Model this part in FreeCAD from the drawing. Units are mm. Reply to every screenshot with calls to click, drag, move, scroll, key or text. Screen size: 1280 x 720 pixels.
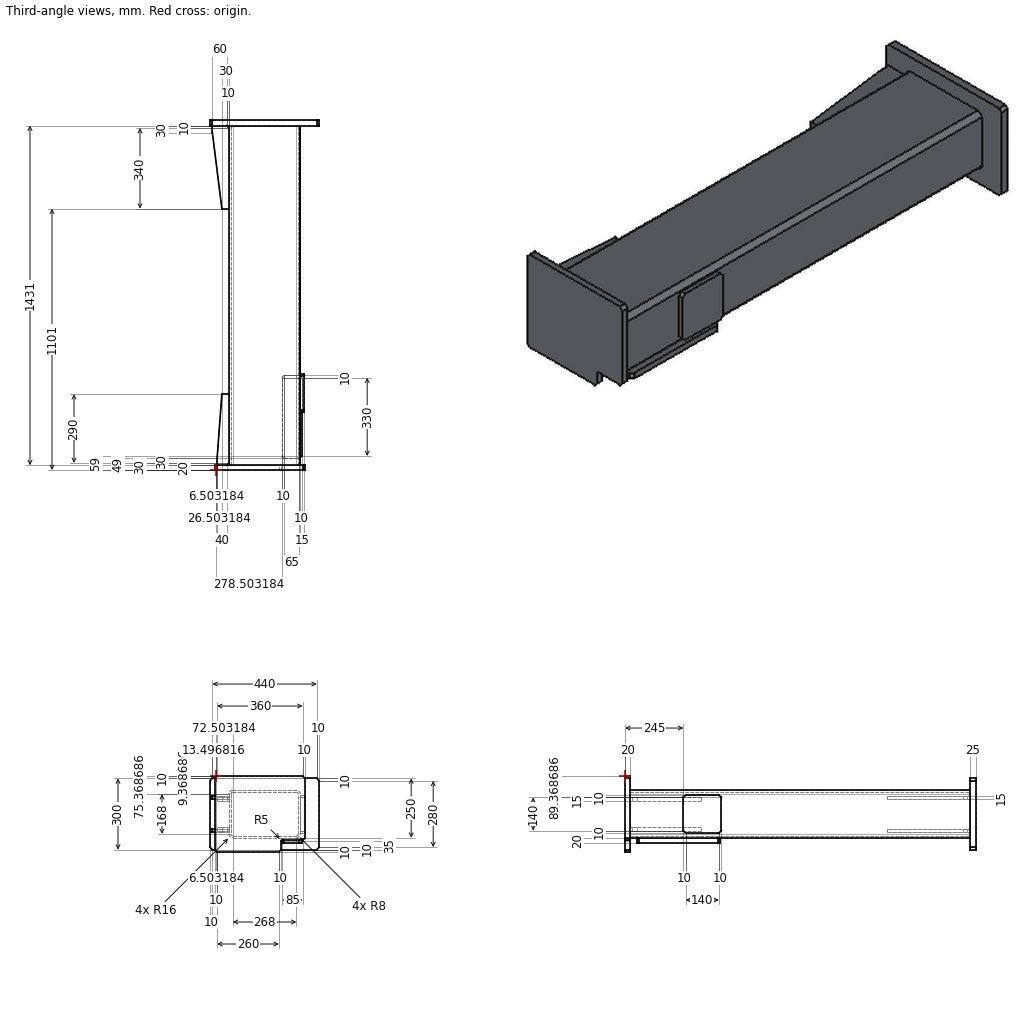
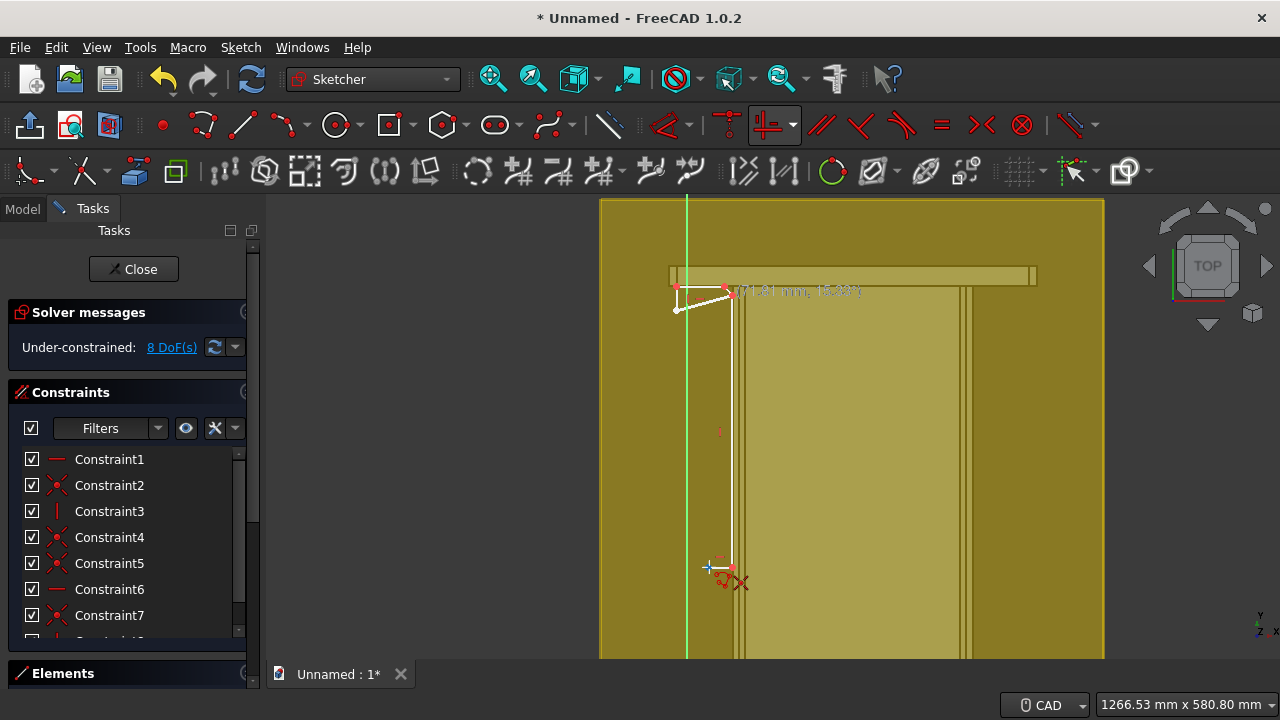
click(708, 568)
key(Escape)
key(Escape)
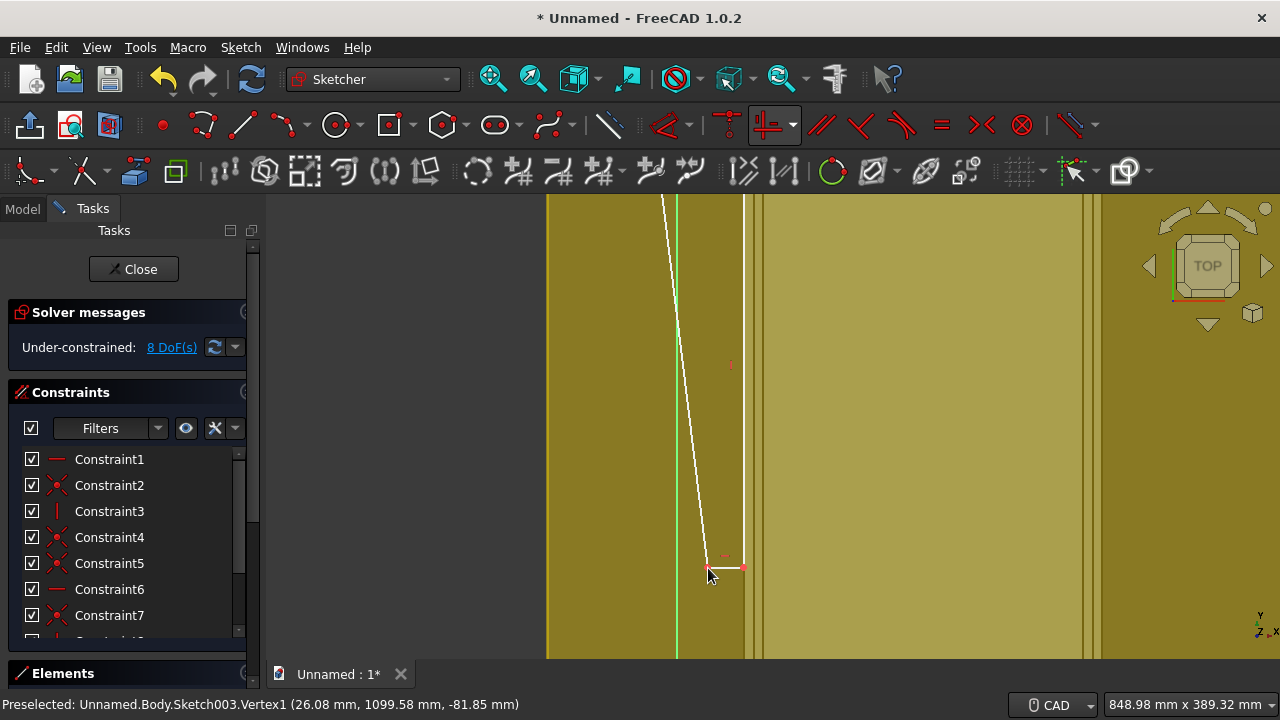
click(664, 126)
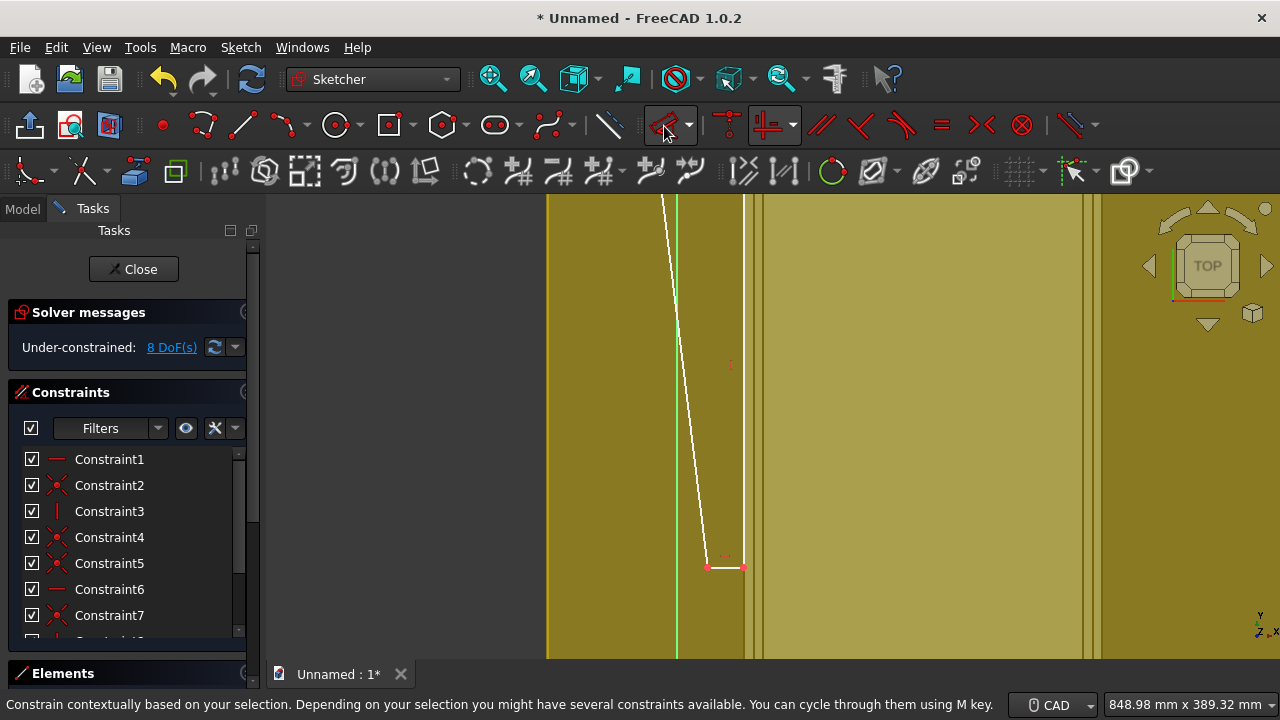
scroll(719, 568, up, 2)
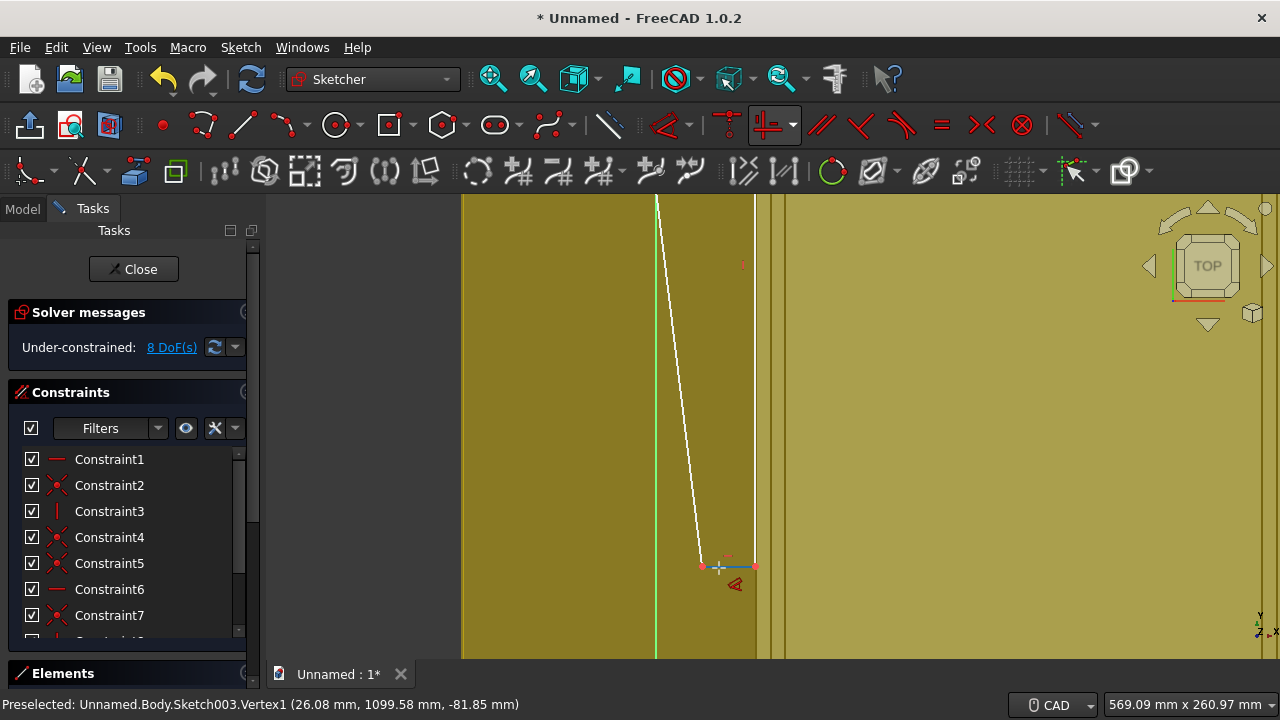
click(718, 567)
click(729, 601)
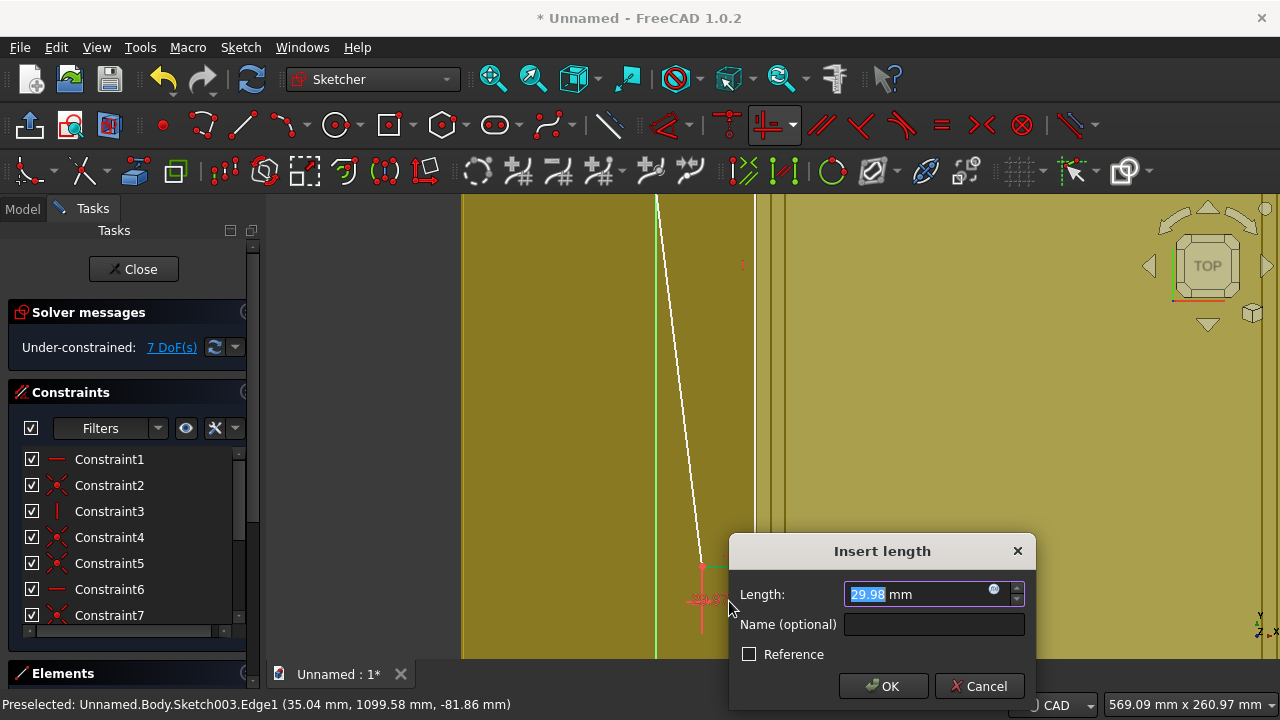
text(30)
key(Return)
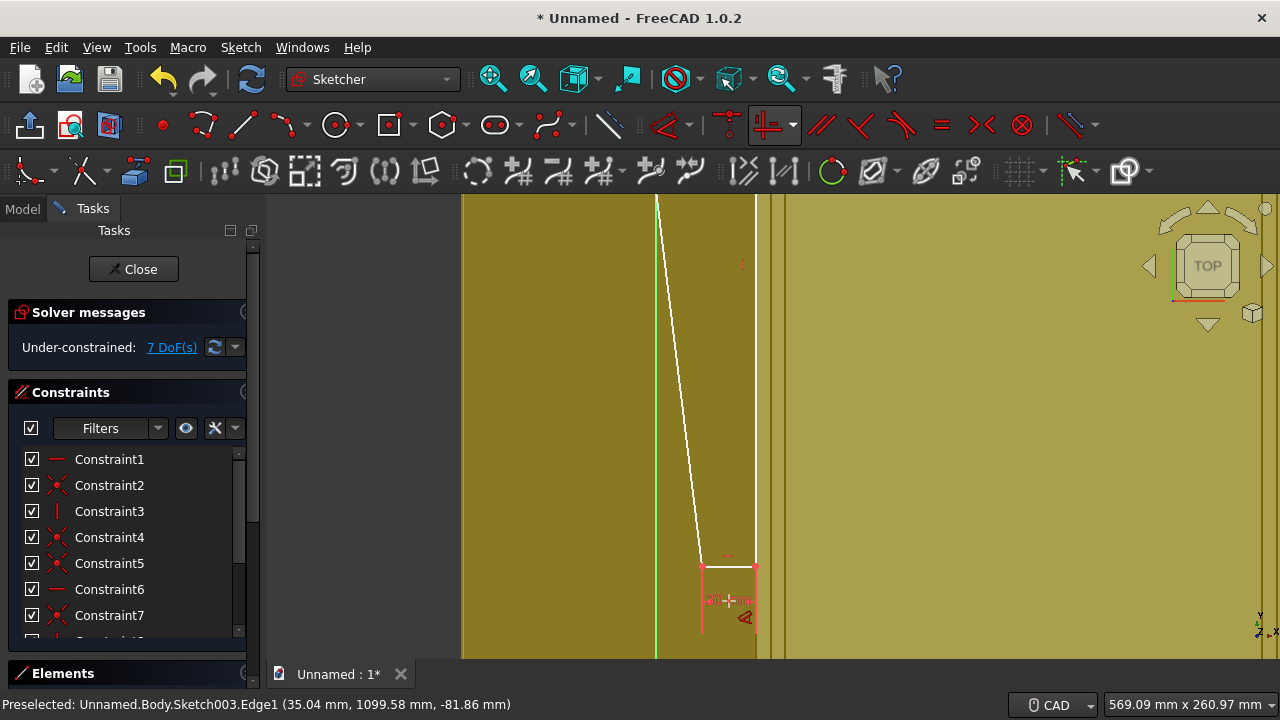
scroll(713, 568, down, 4)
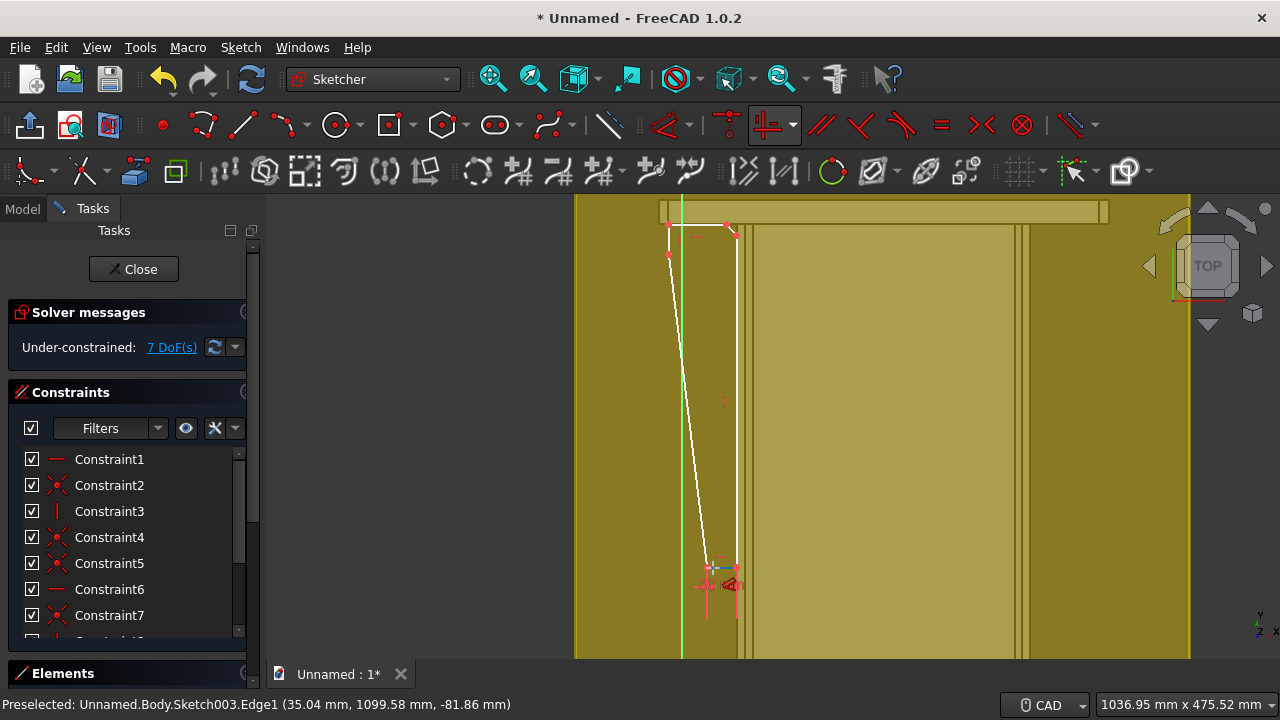
click(710, 287)
click(701, 253)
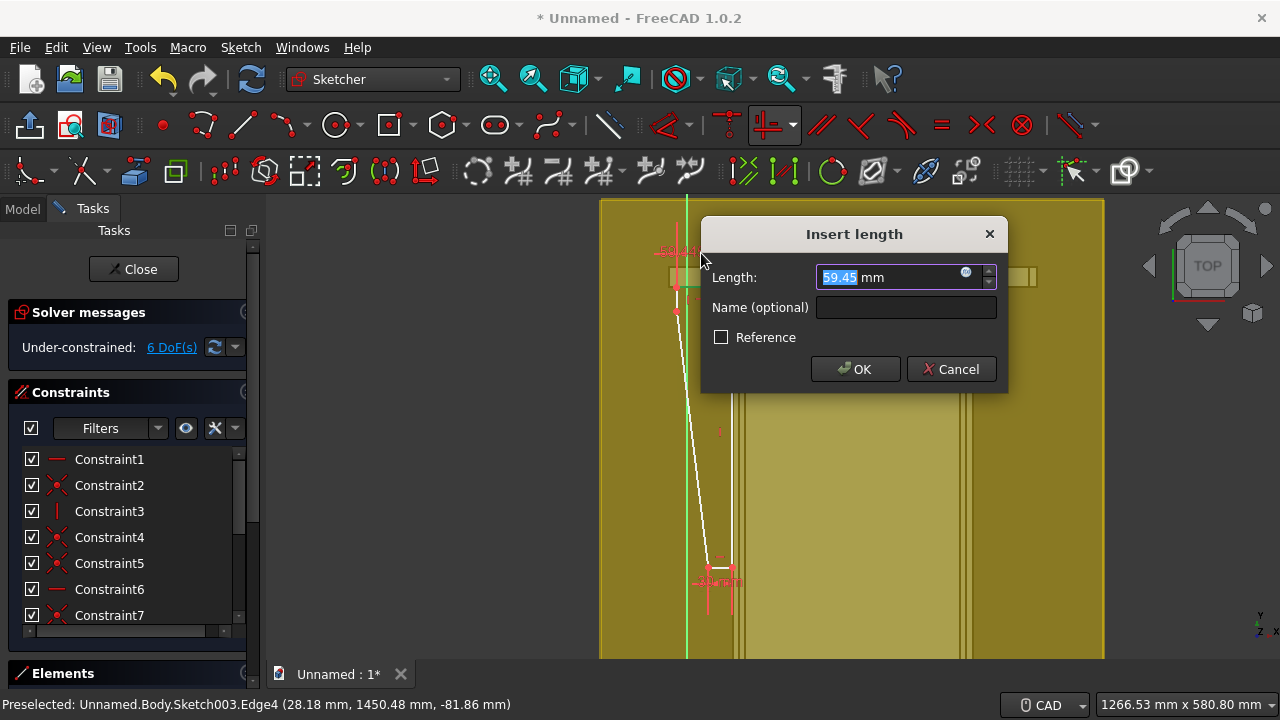
text(60)
key(Return)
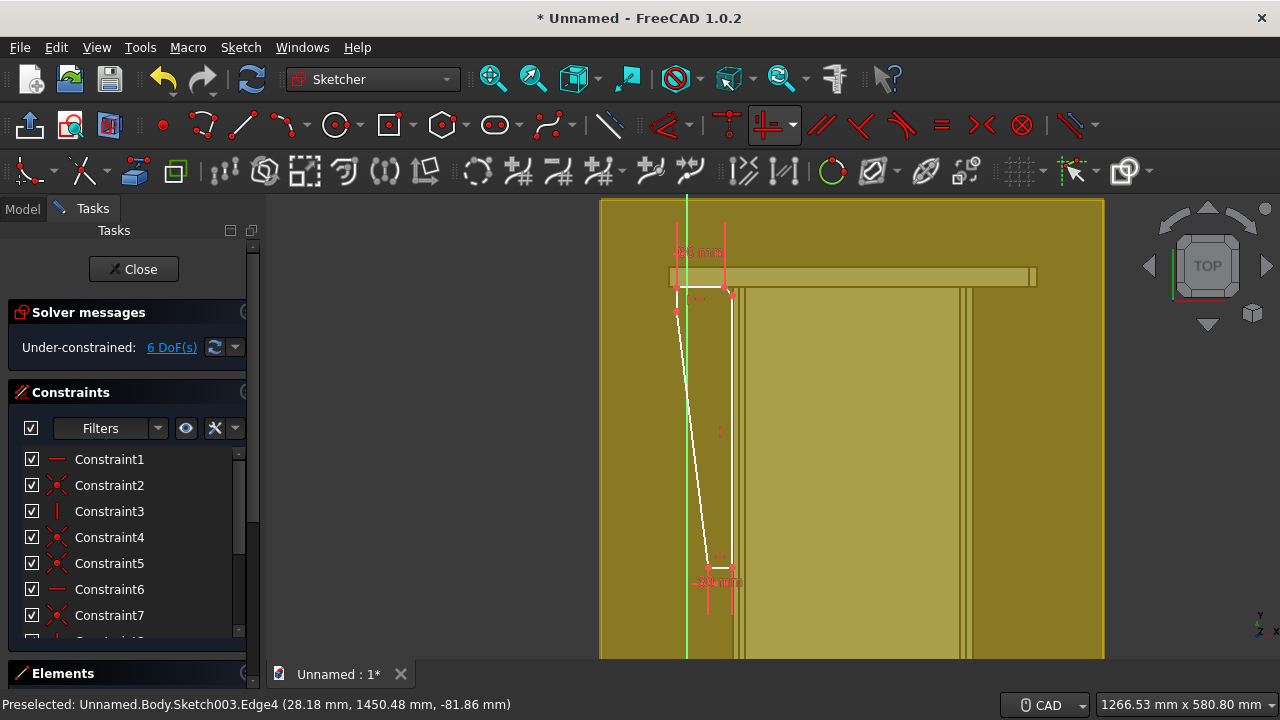
scroll(677, 297, up, 3)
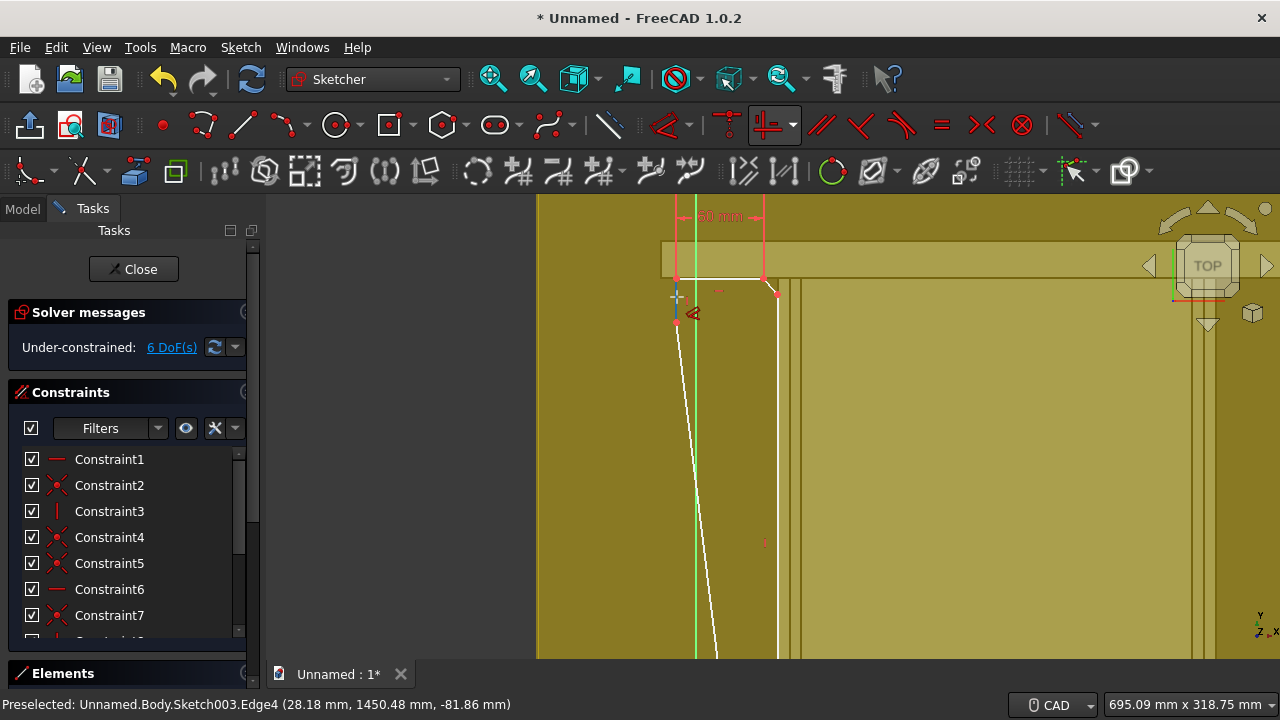
click(676, 296)
click(642, 301)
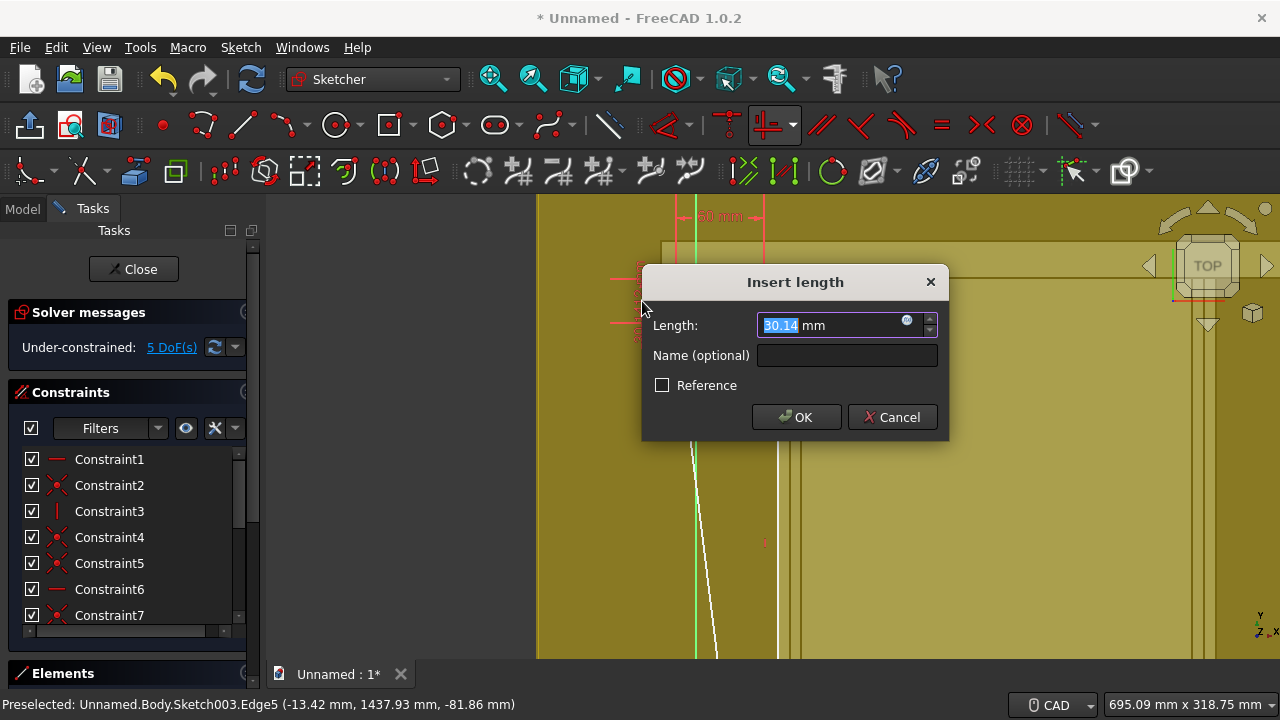
text(30)
key(Return)